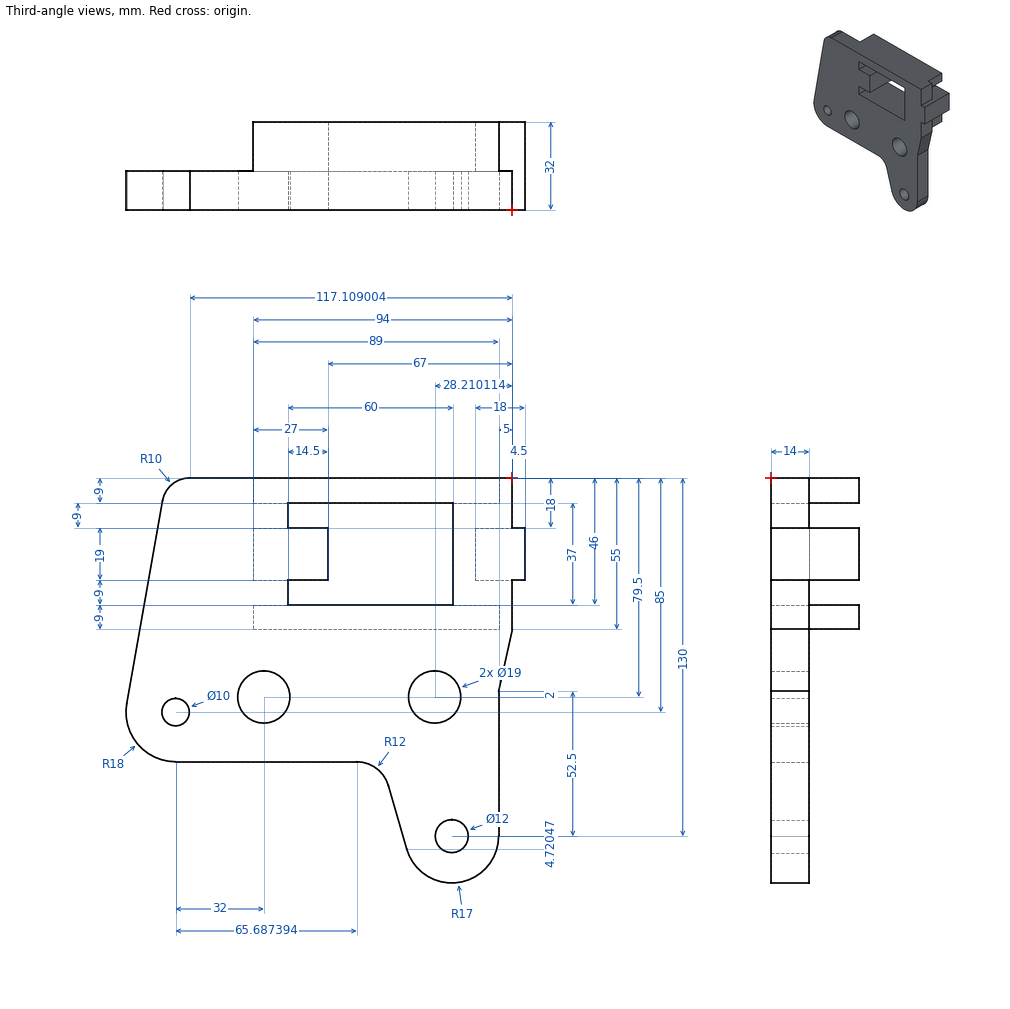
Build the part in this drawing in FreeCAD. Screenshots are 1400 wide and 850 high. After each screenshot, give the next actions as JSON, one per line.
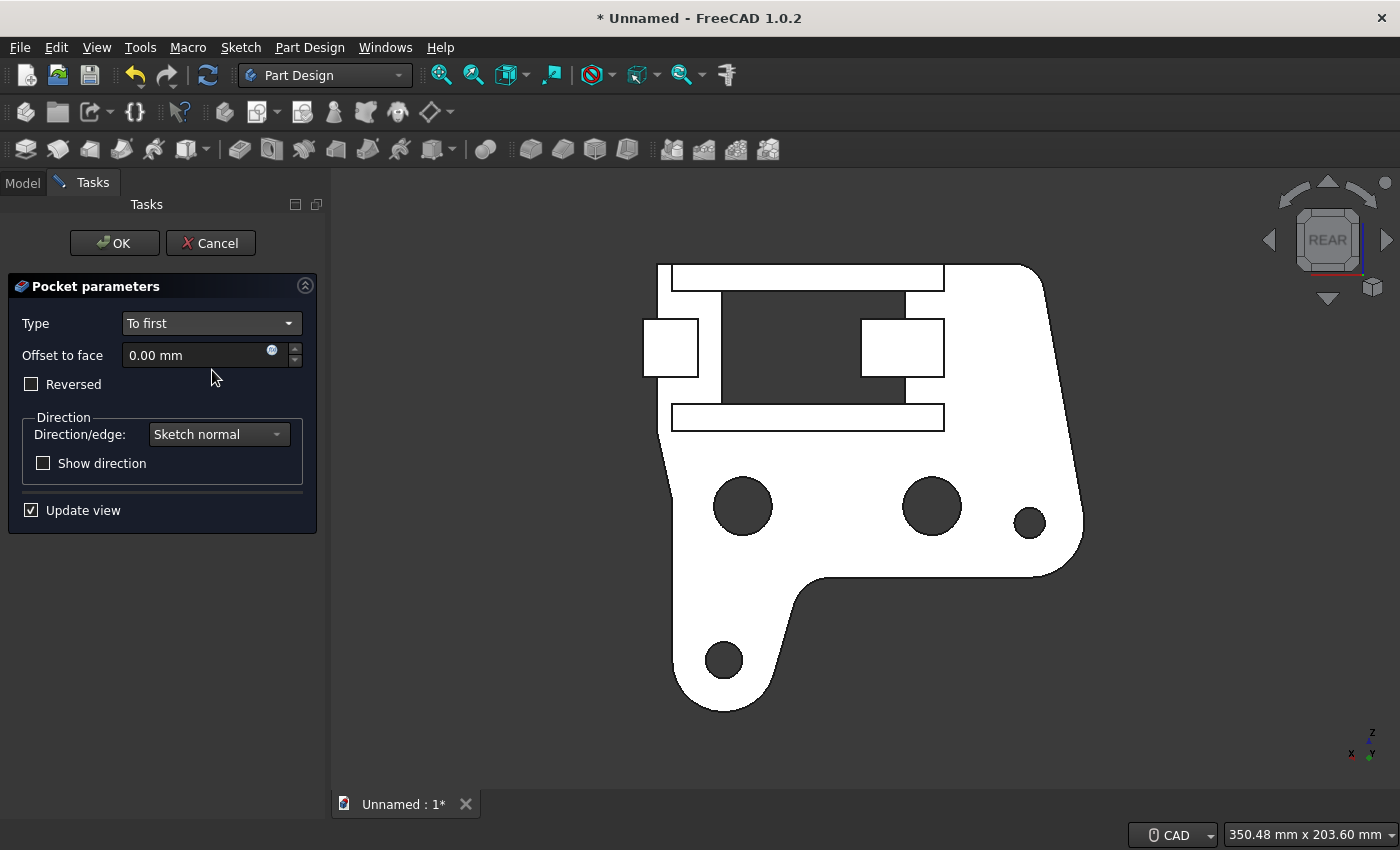
{"action": "left_click", "coordinate": [115, 243]}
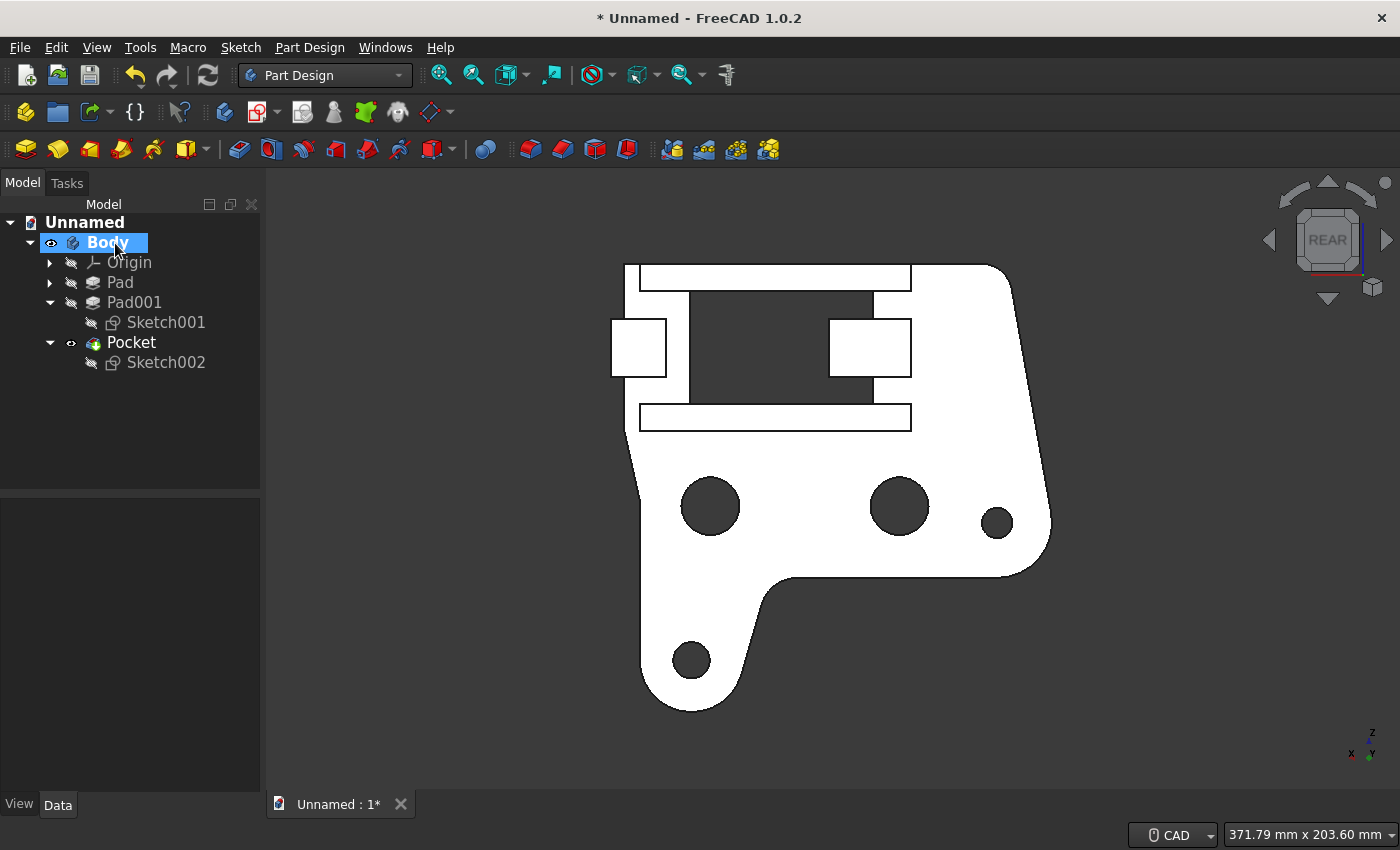
{"action": "key", "text": "0"}